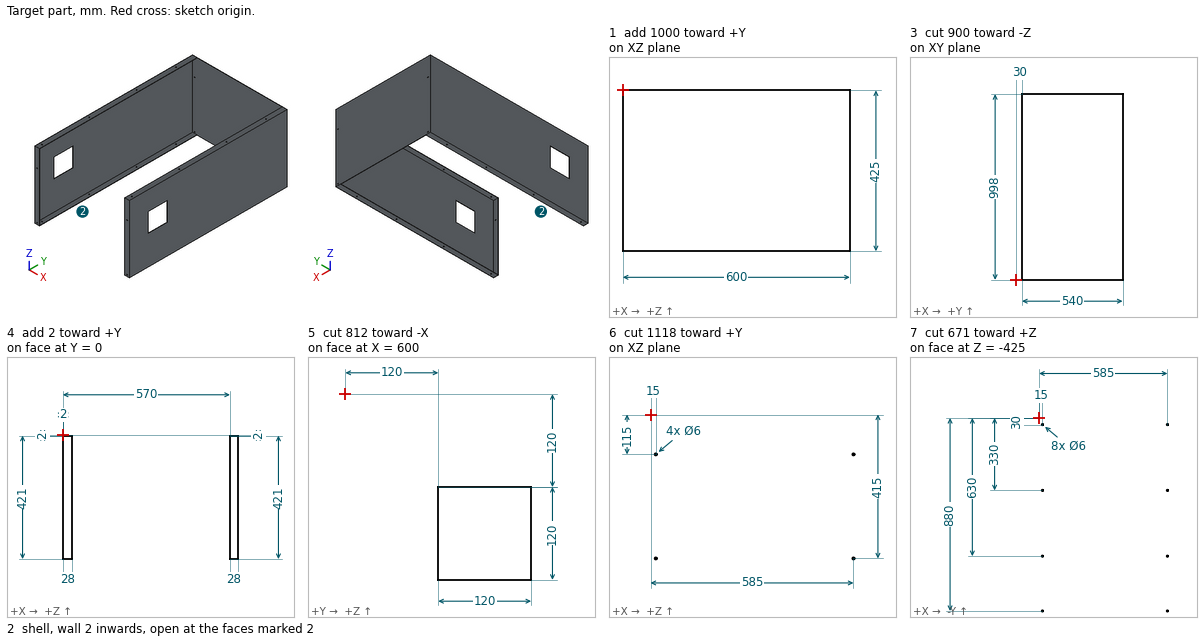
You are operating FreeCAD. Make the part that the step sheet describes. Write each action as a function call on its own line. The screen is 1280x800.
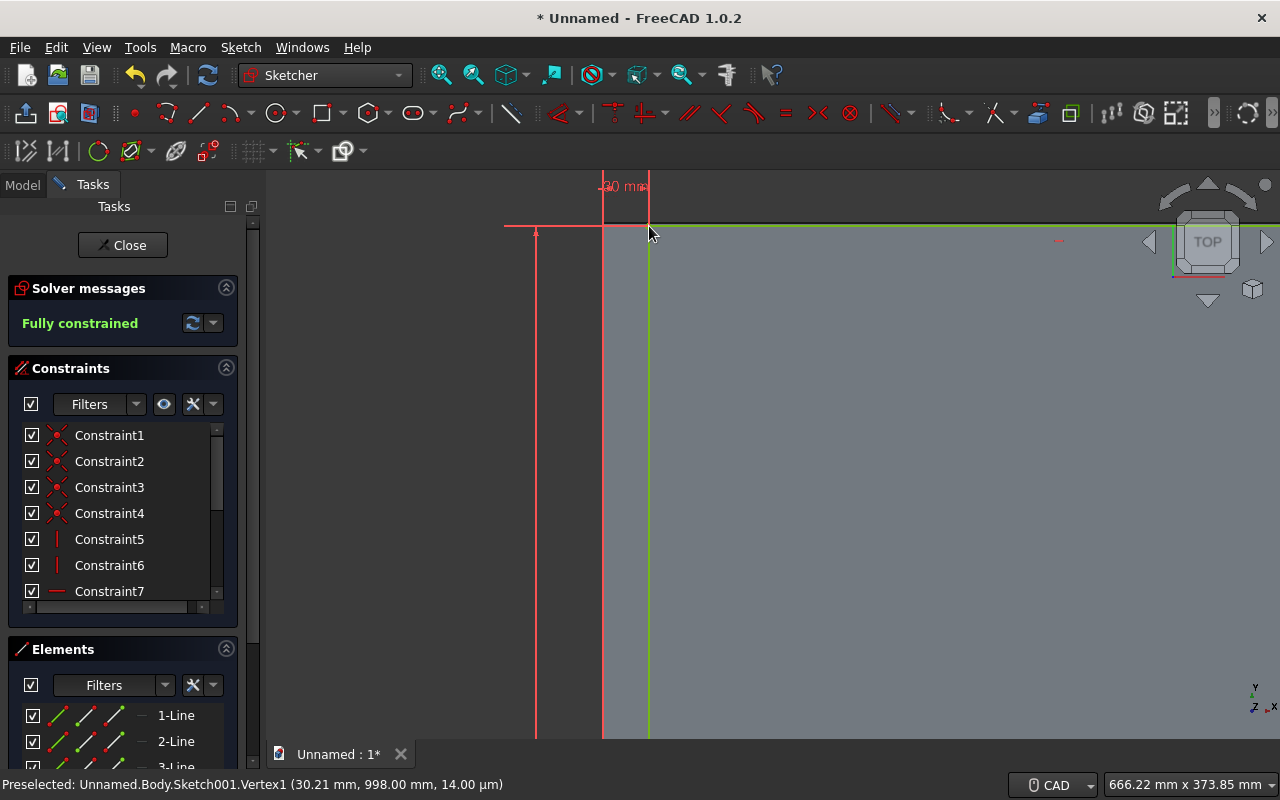
click(123, 245)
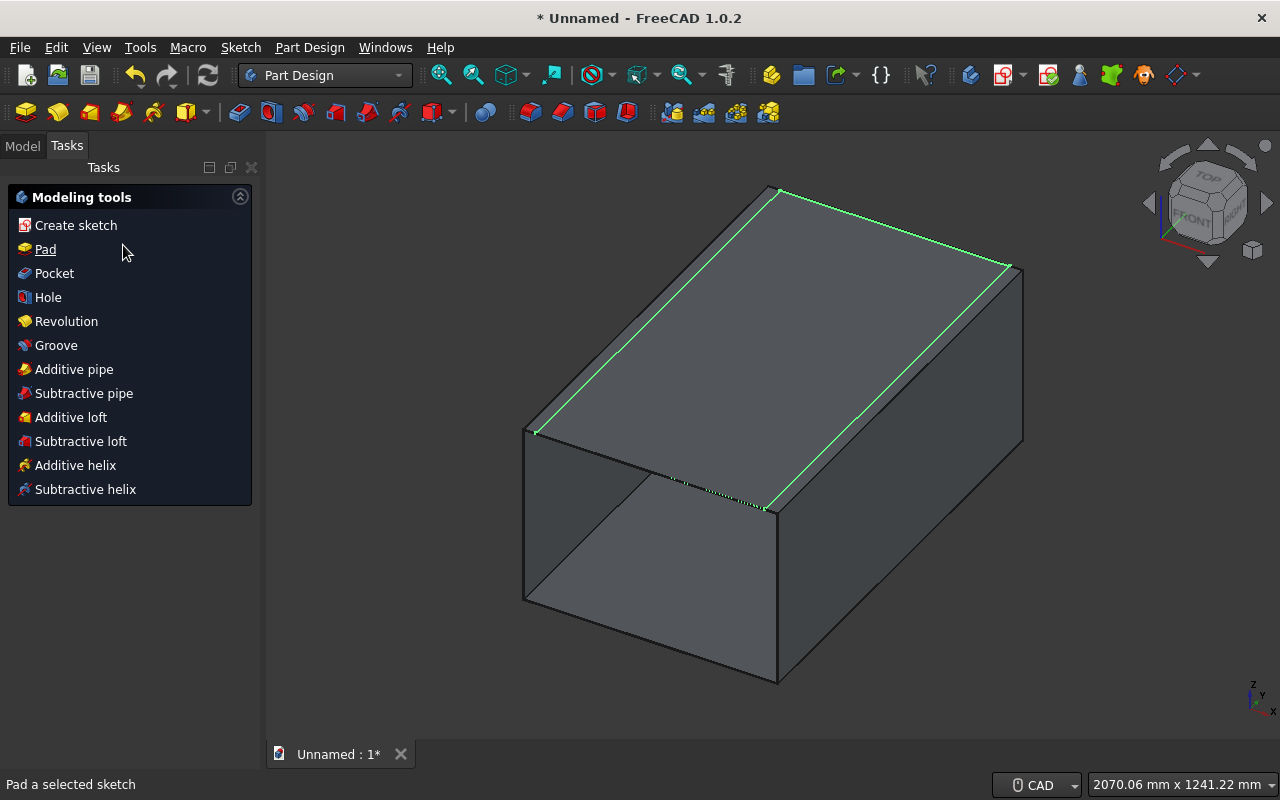
click(240, 112)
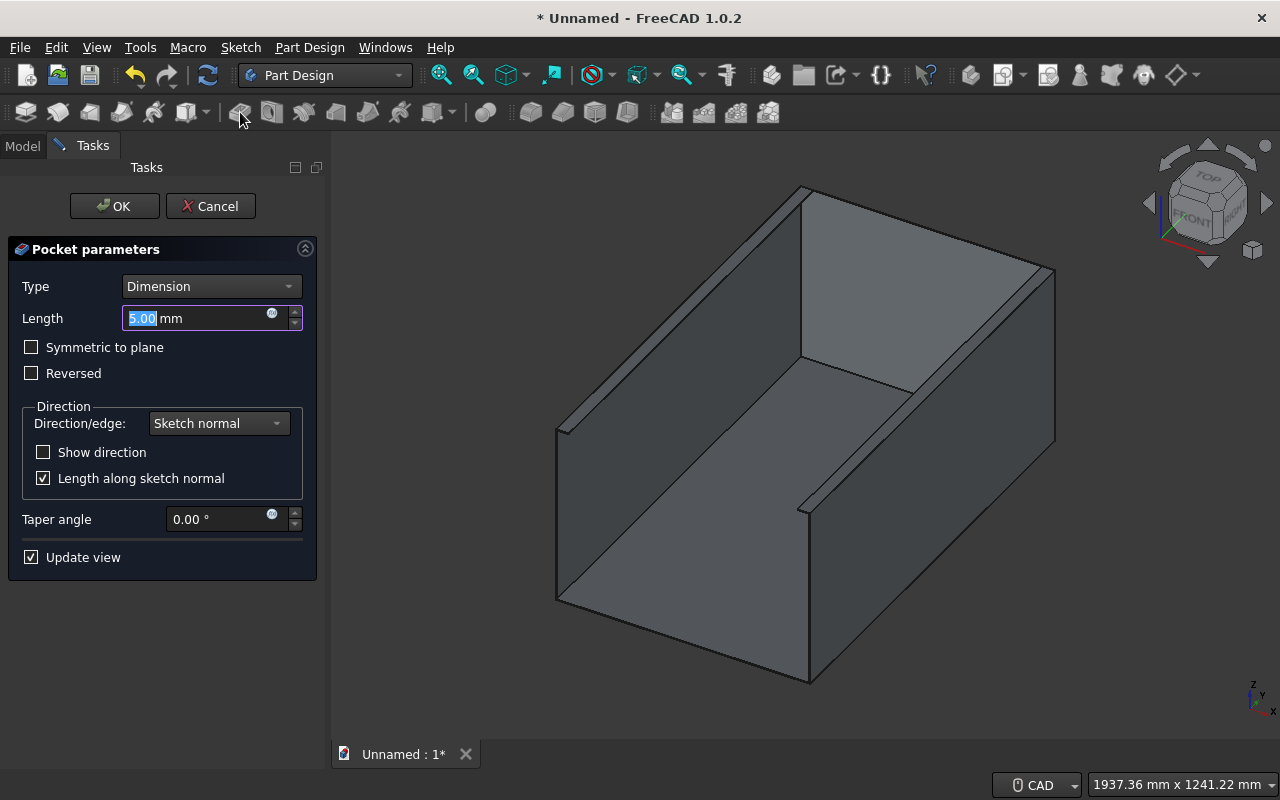
text(900)
key(Tab)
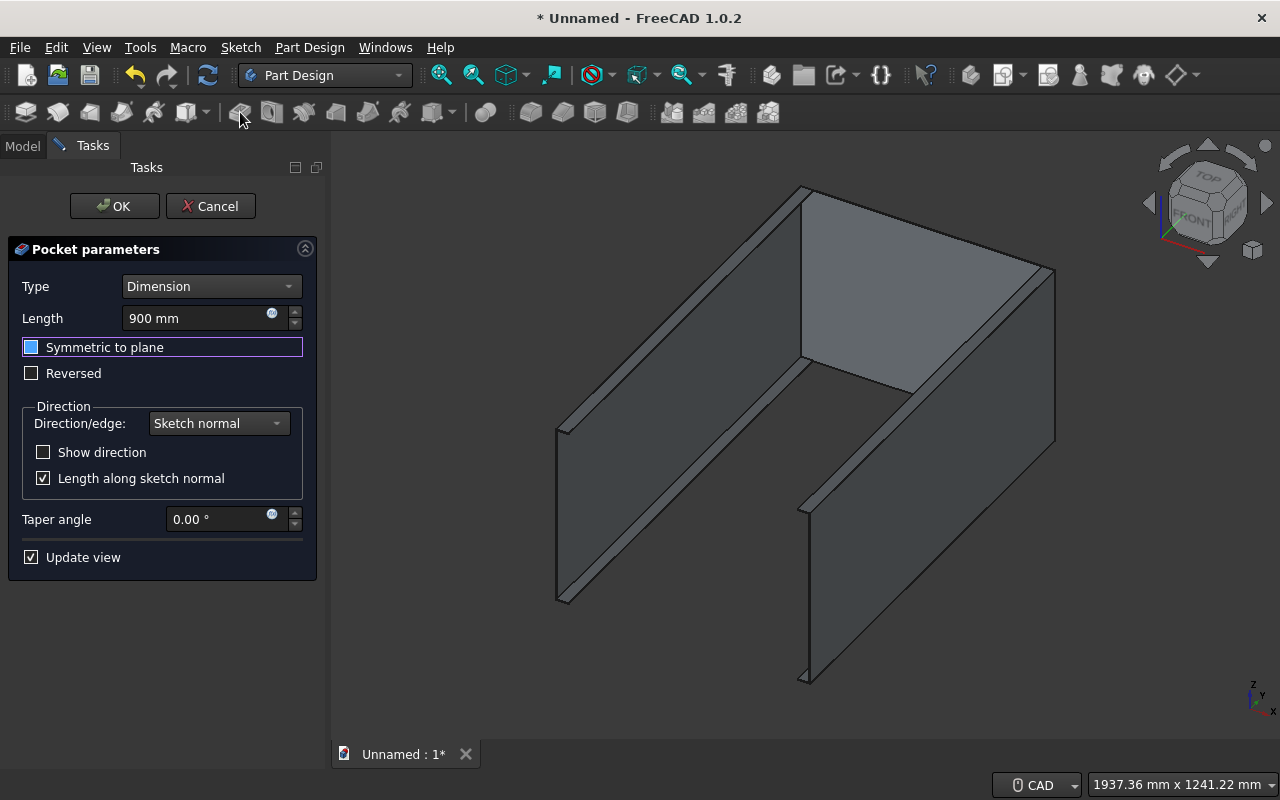
click(115, 206)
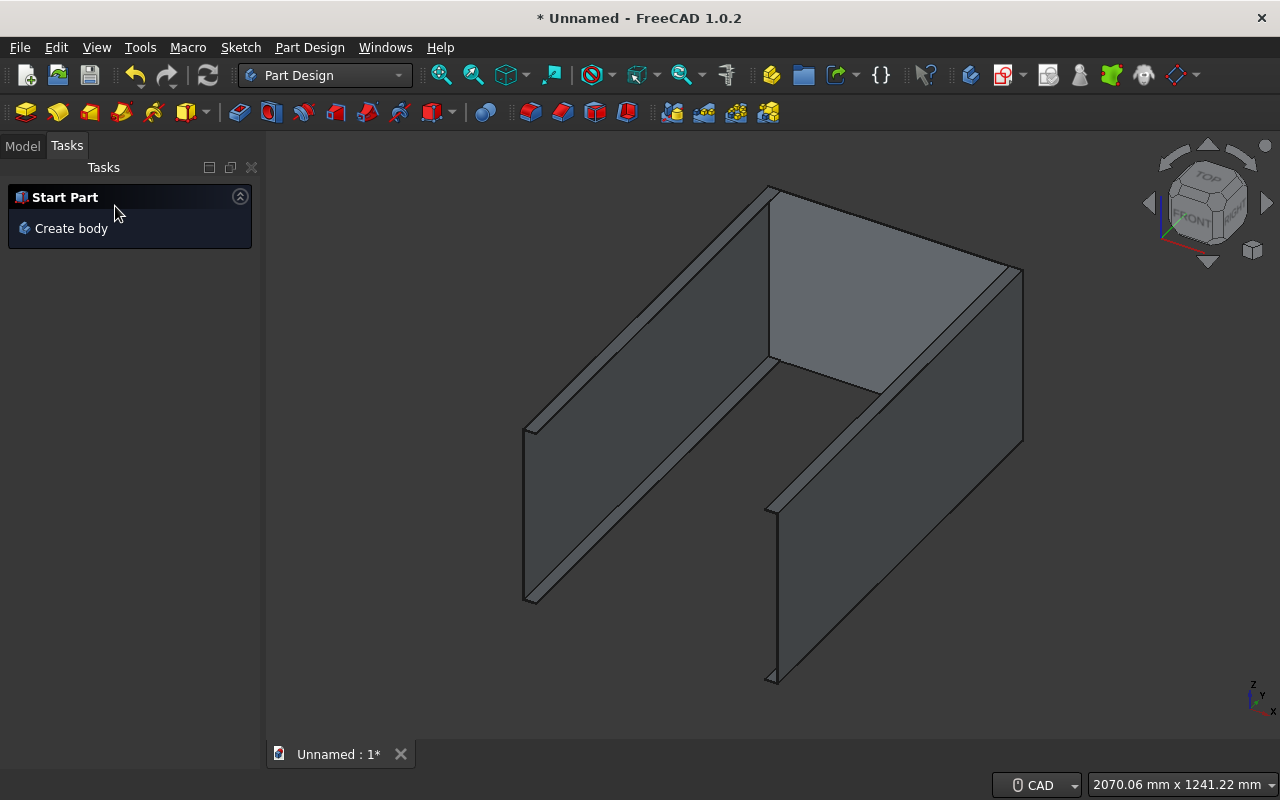
scroll(777, 569, up, 15)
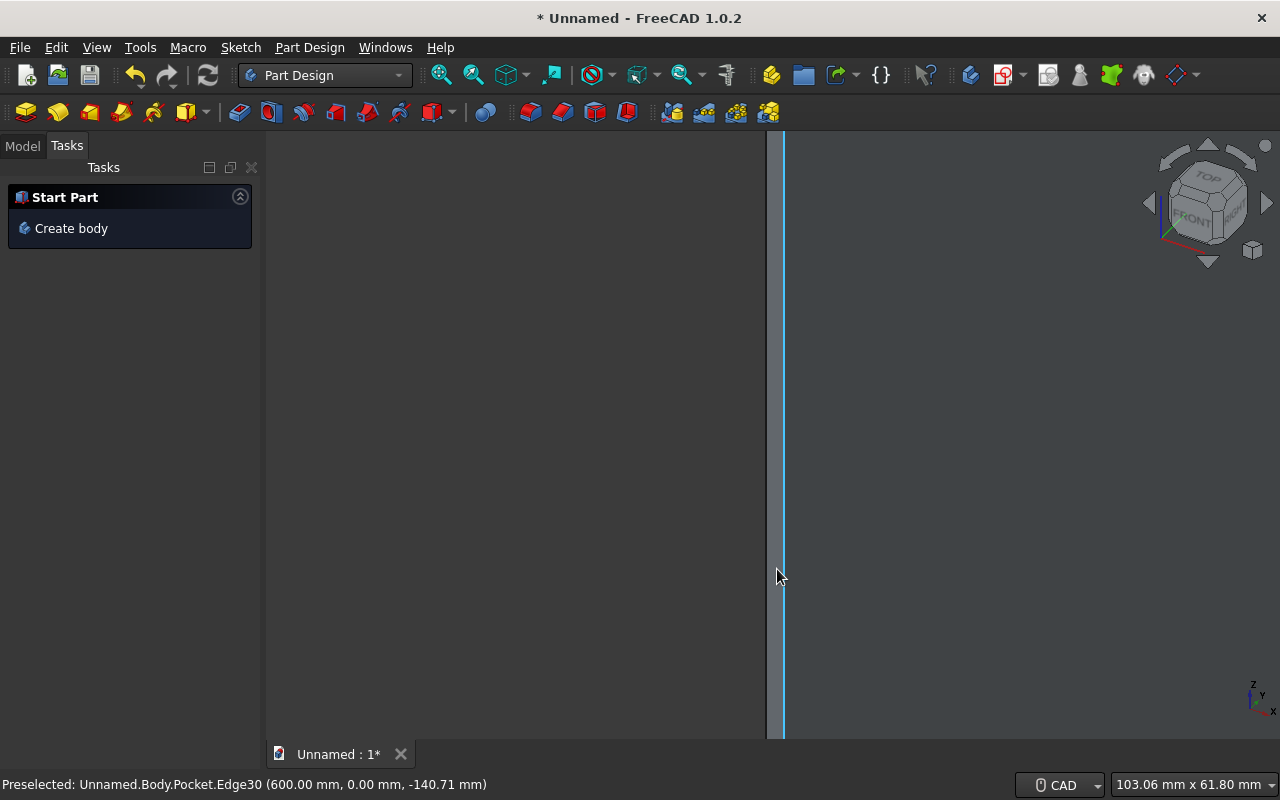
click(772, 578)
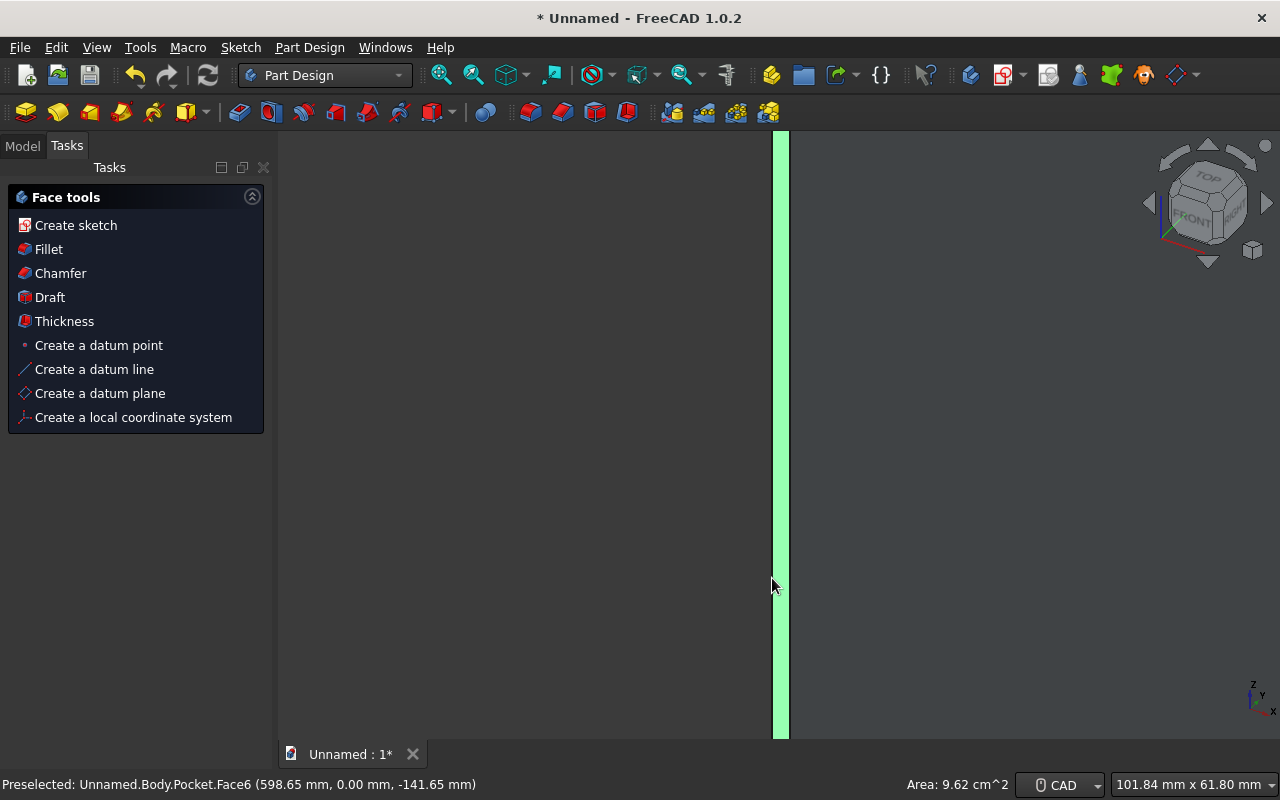
click(1004, 76)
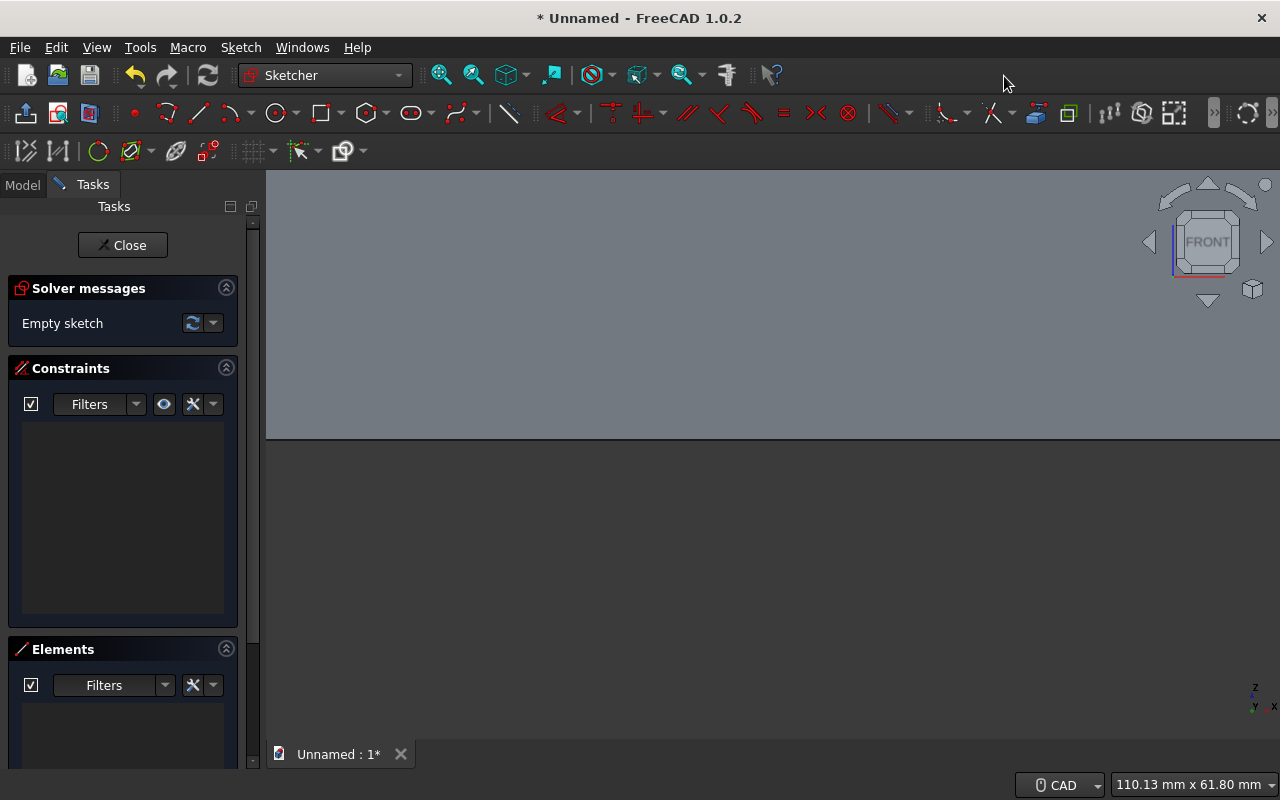
scroll(774, 652, down, 12)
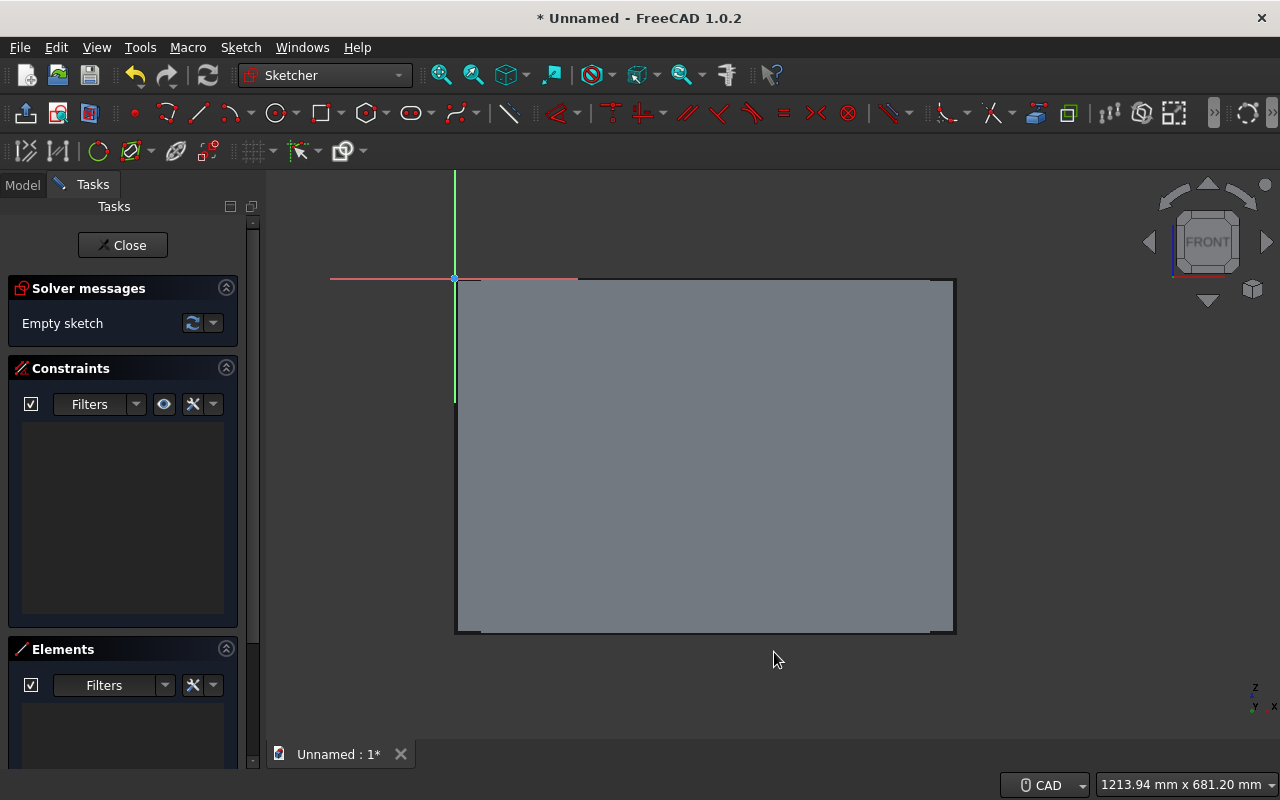
click(322, 114)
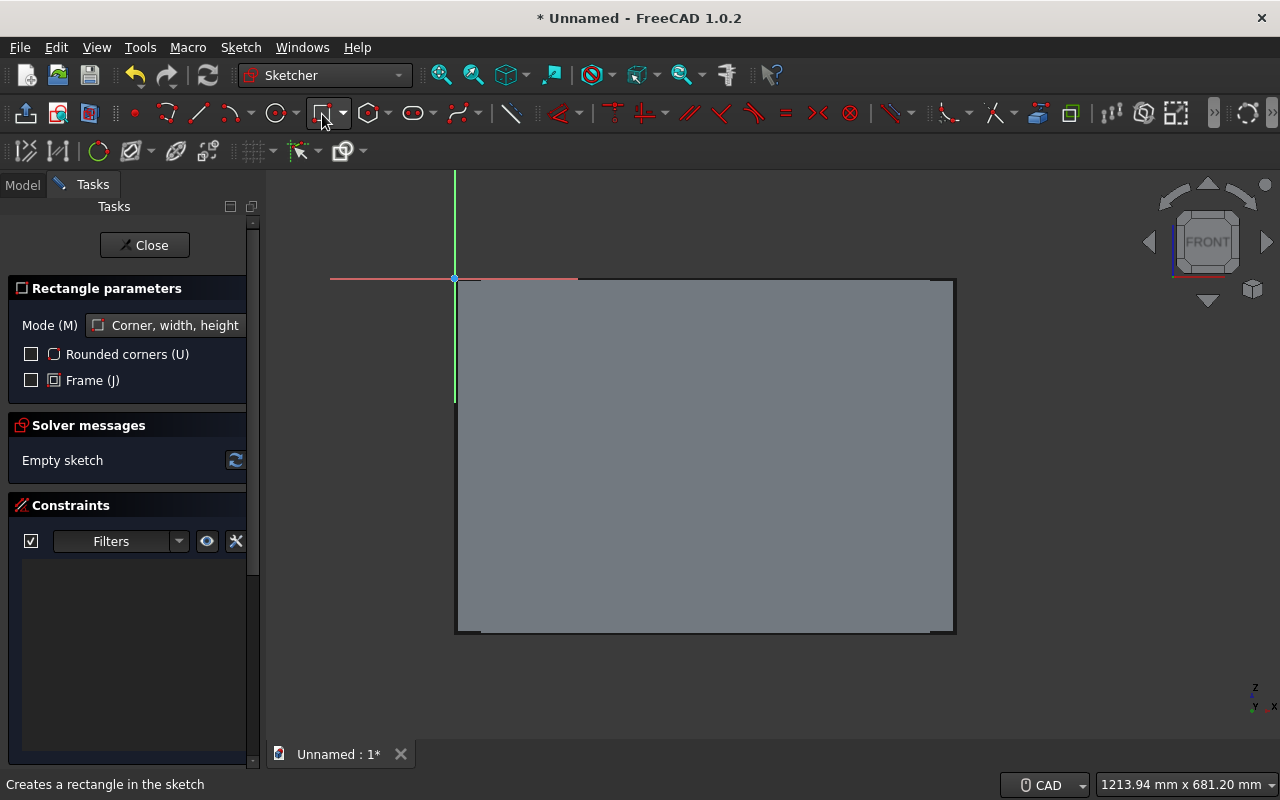
scroll(457, 280, up, 12)